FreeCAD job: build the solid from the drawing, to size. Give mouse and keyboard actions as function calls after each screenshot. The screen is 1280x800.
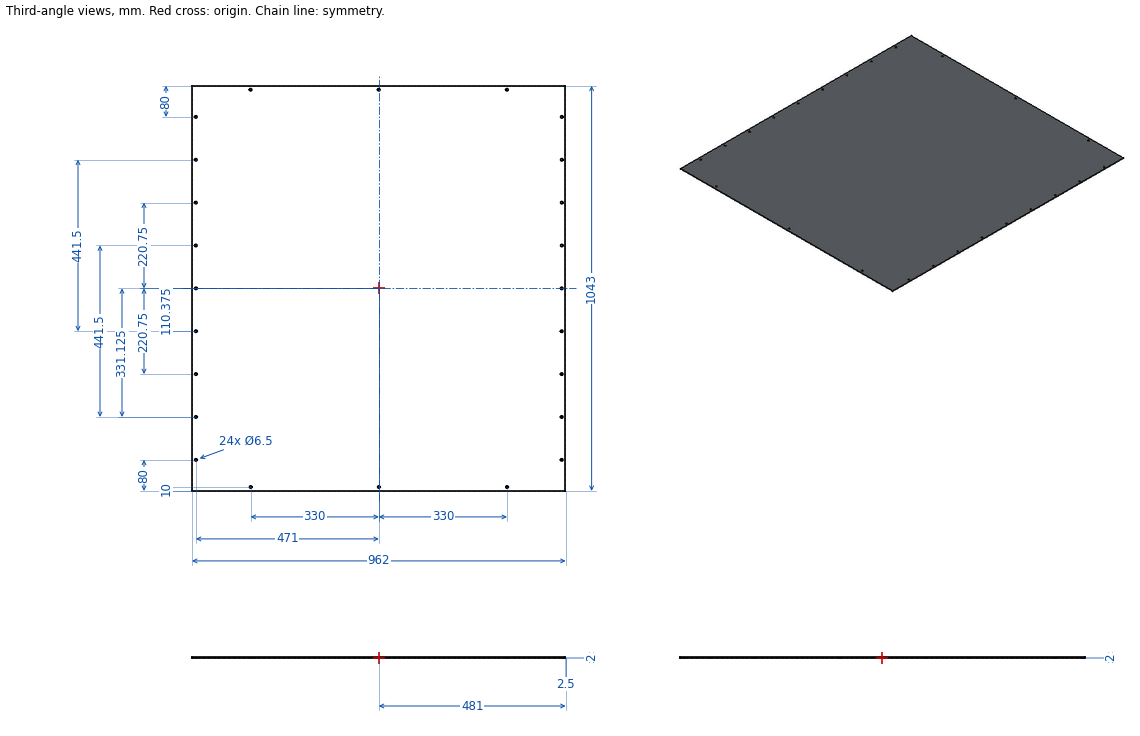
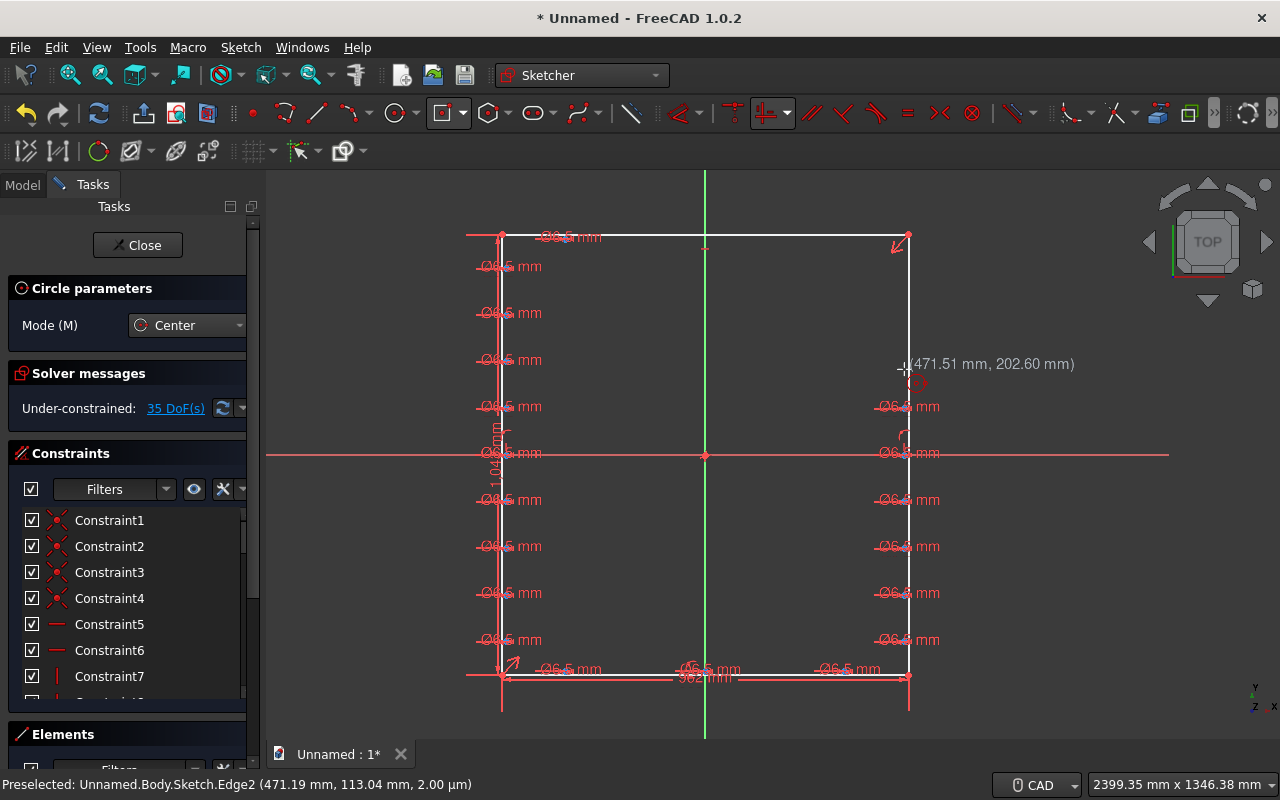
scroll(904, 362, up, 7)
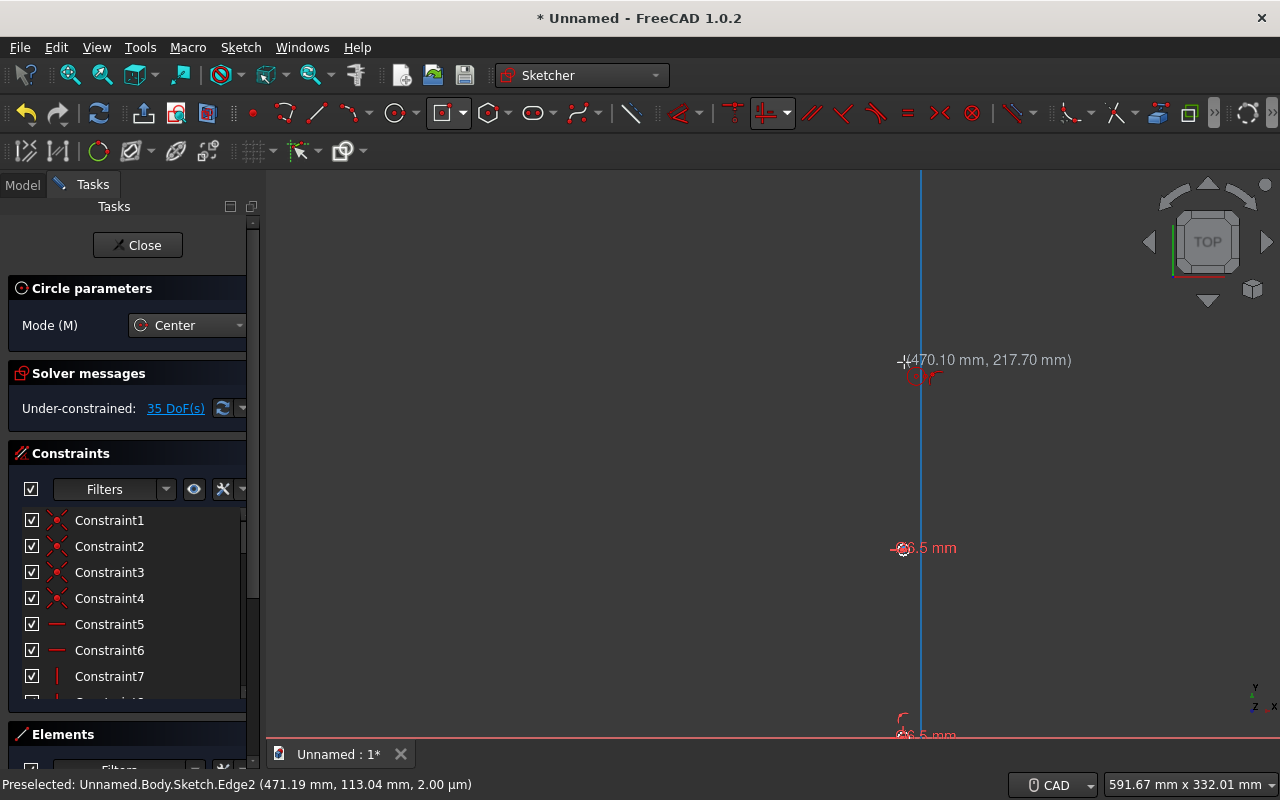
click(904, 360)
move(900, 356)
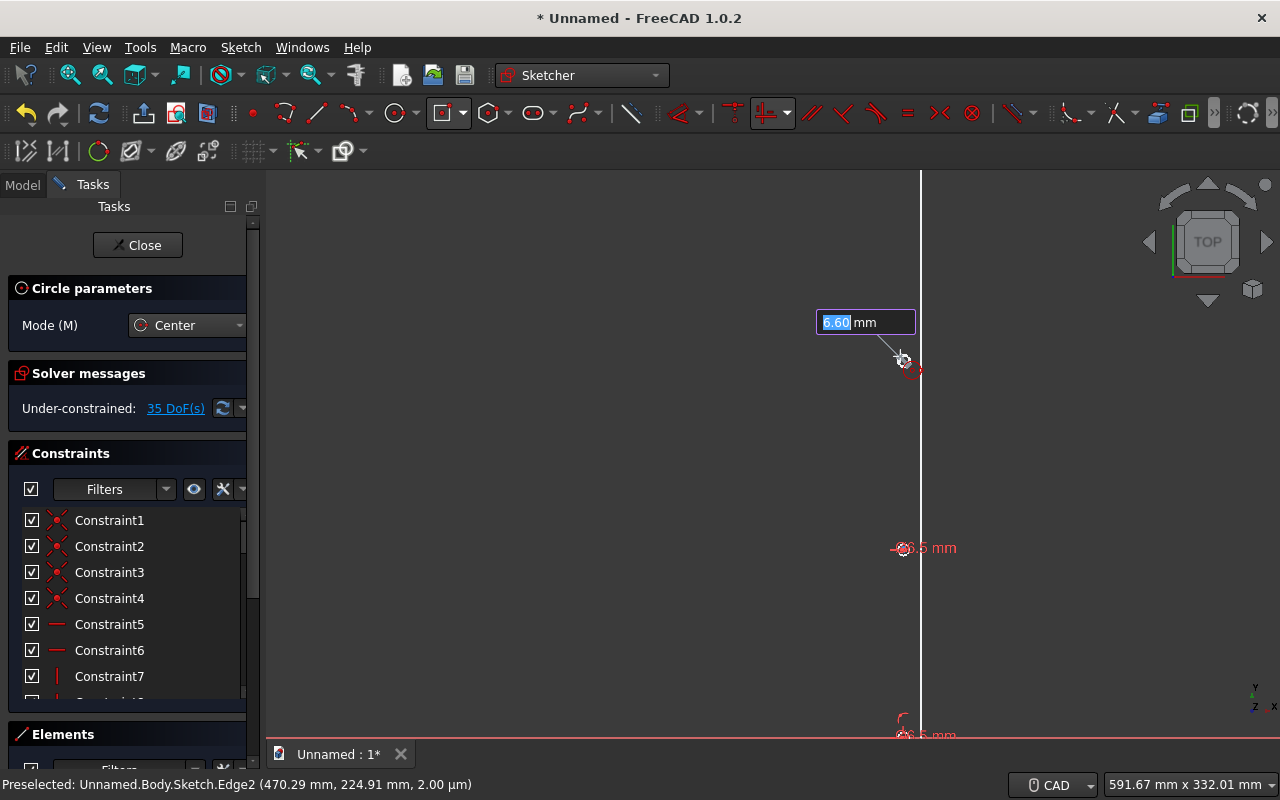
text(6.5)
key(Return)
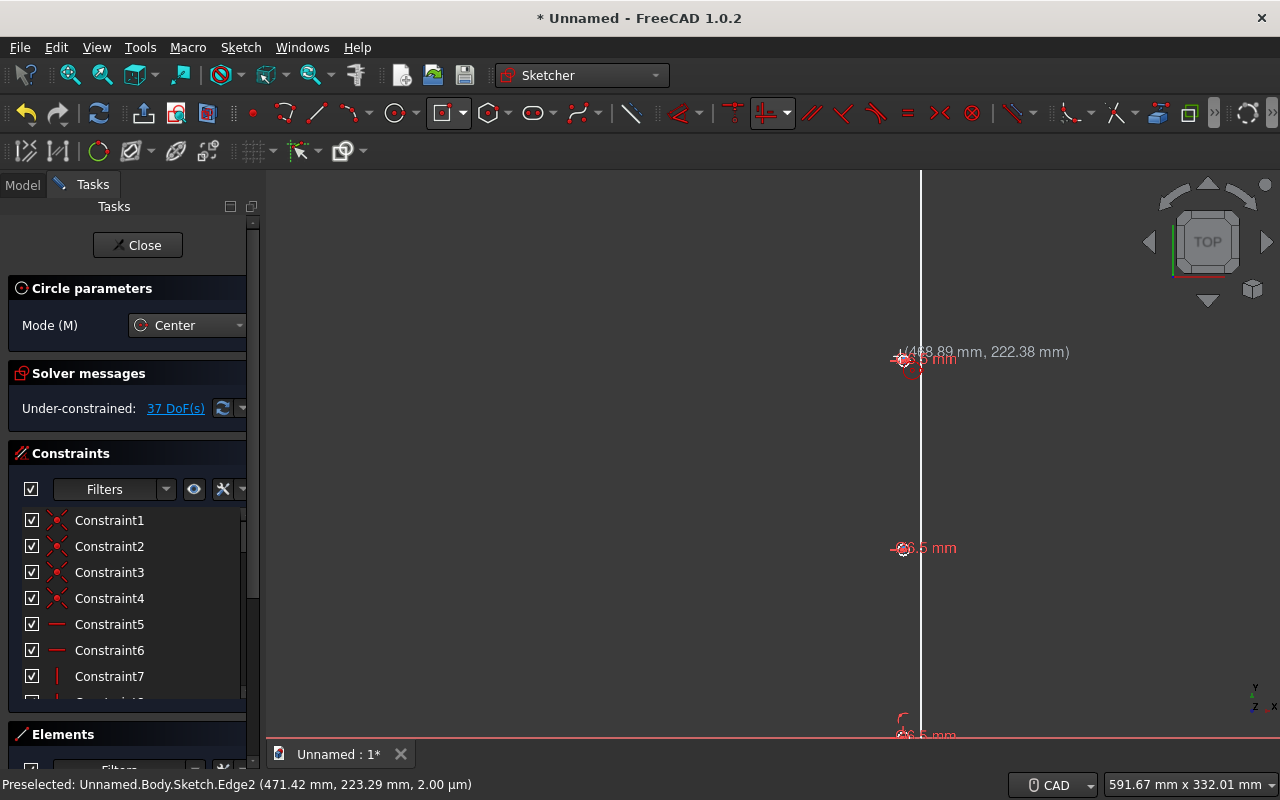
scroll(858, 383, down, 8)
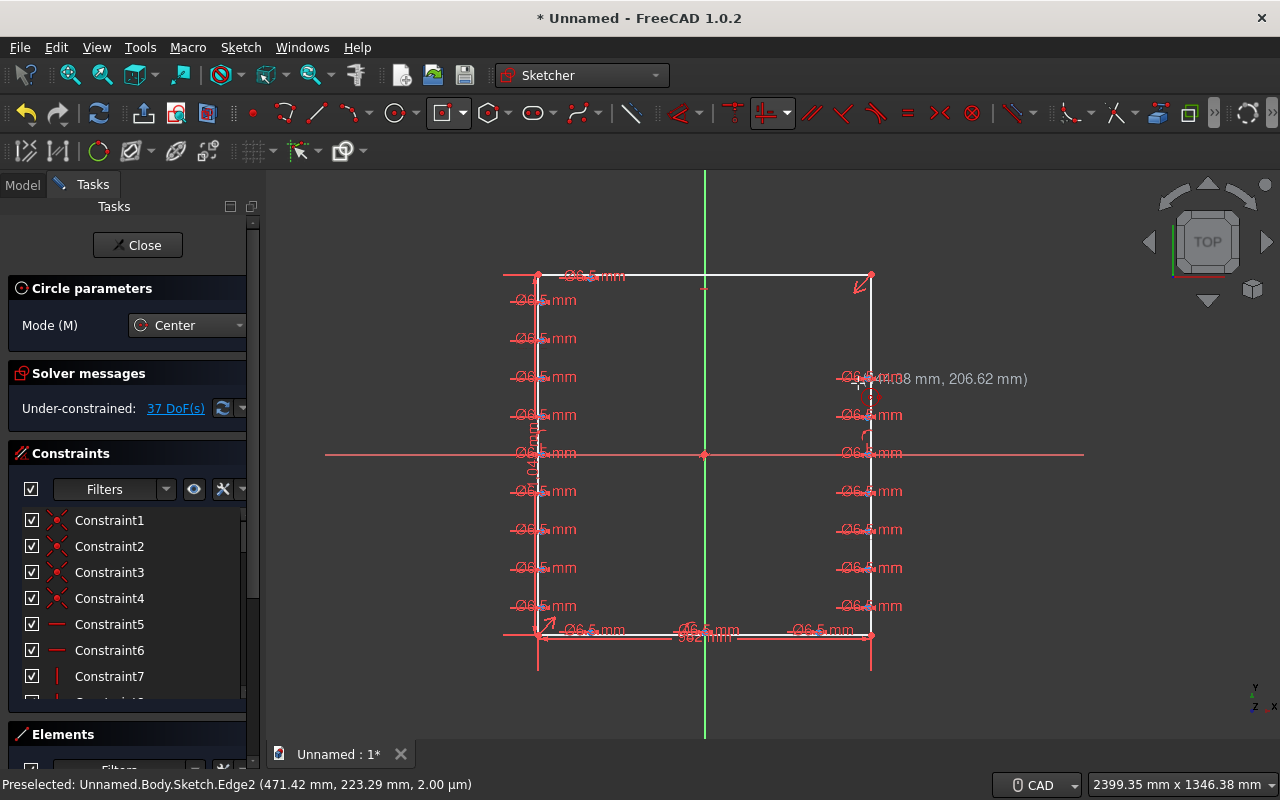
scroll(705, 278, up, 16)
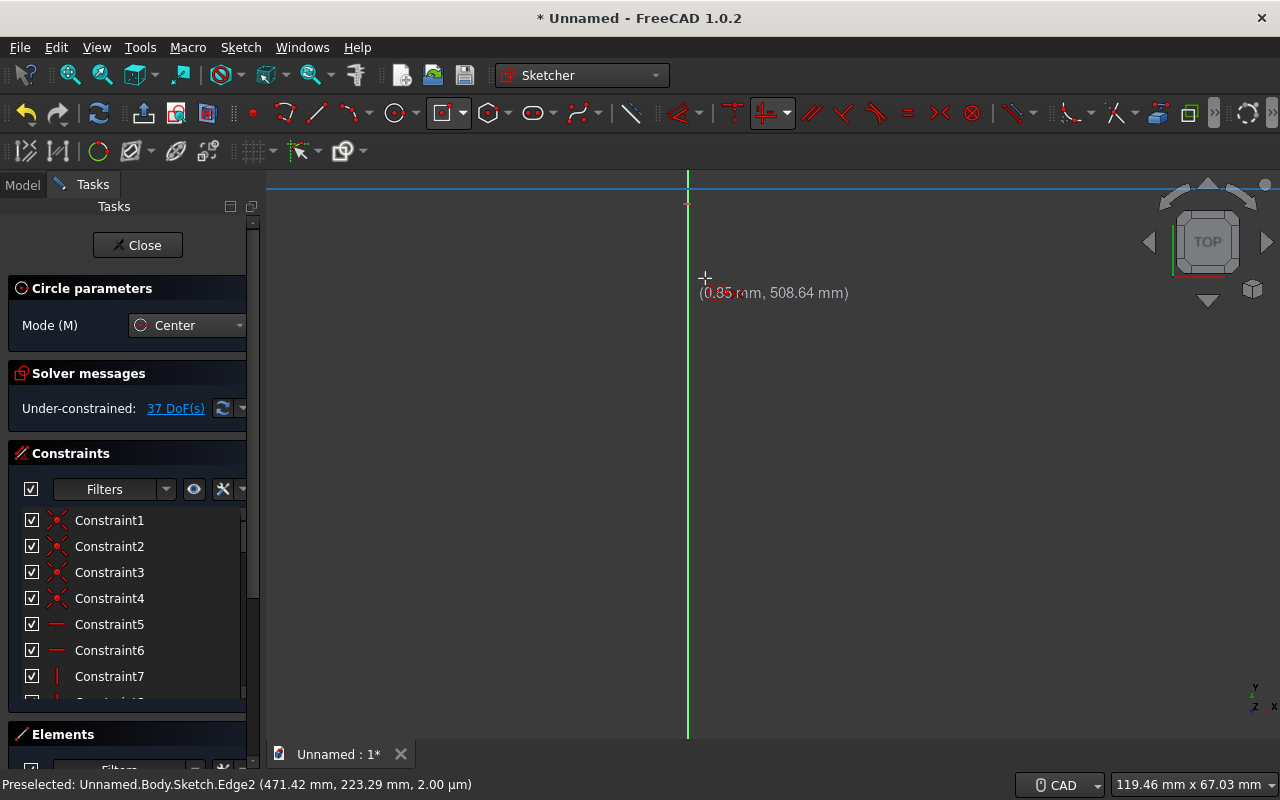
scroll(705, 236, down, 15)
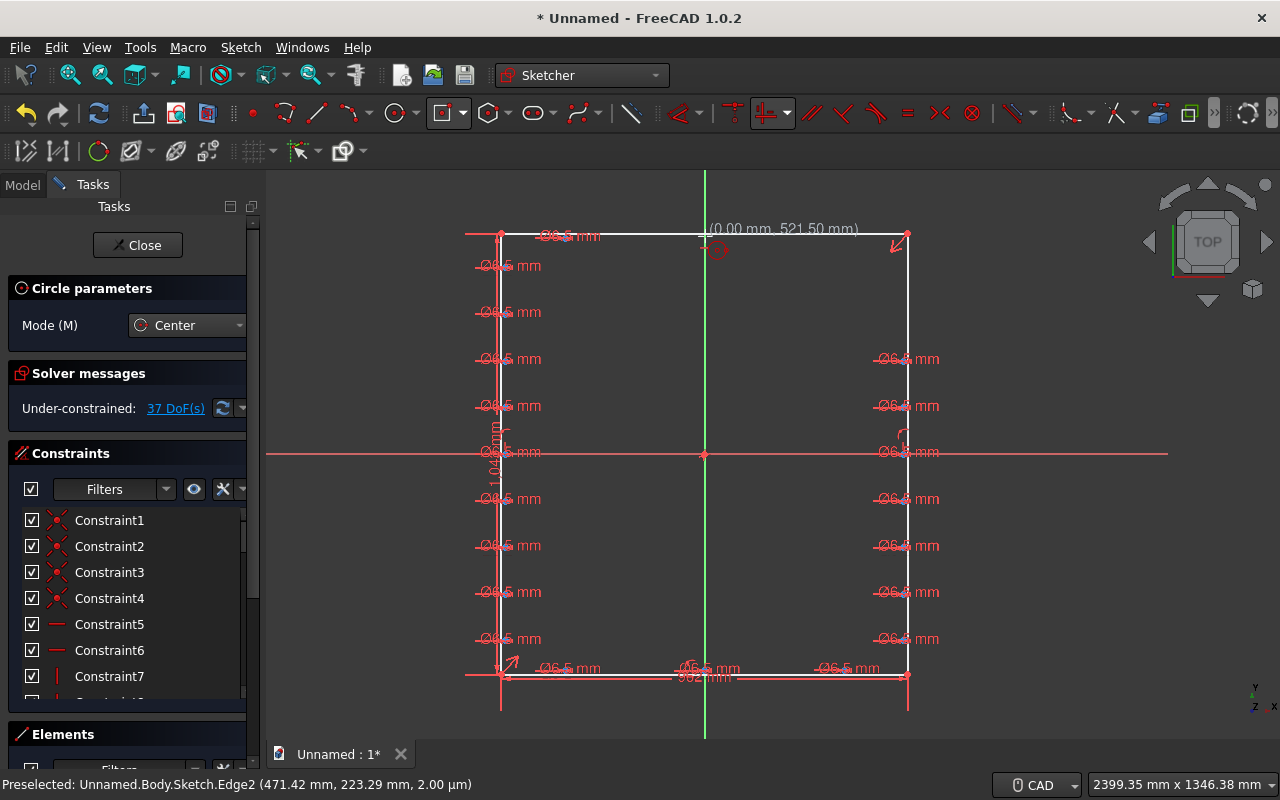
scroll(705, 238, up, 7)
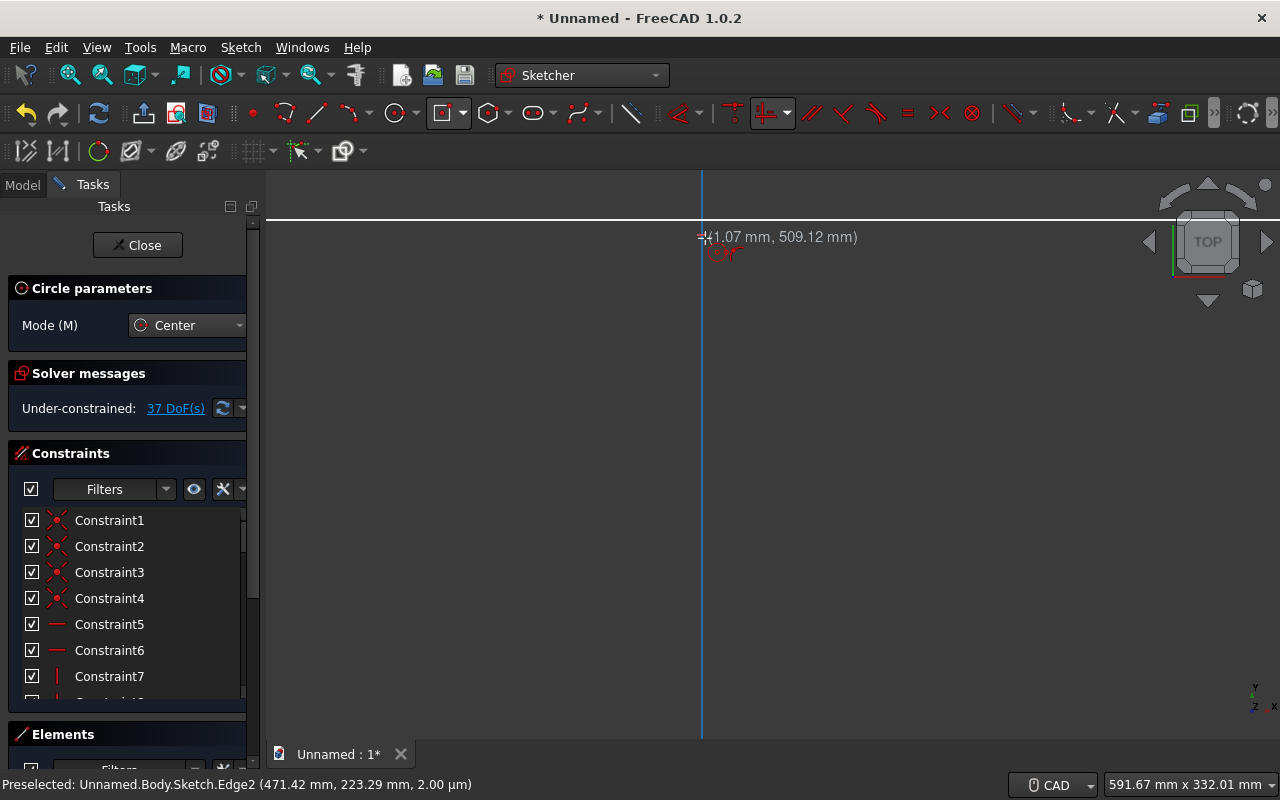
click(702, 238)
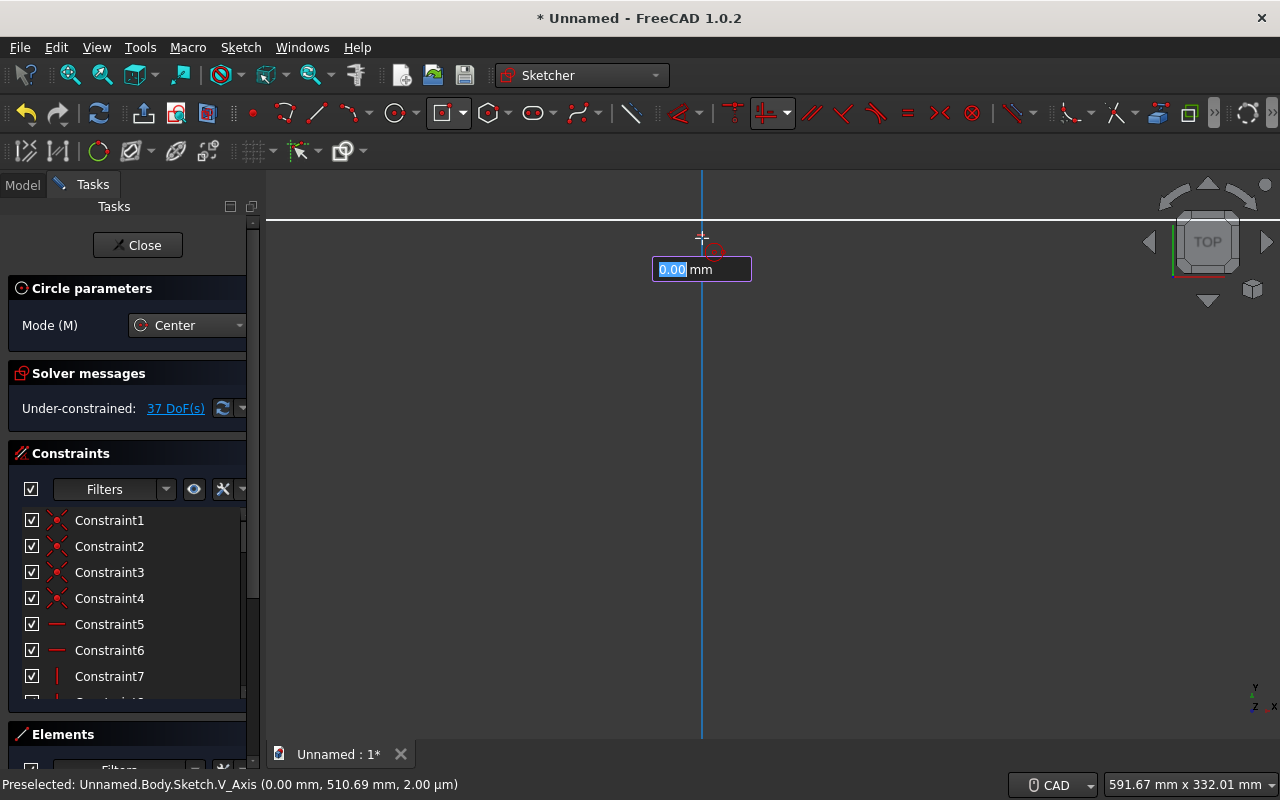
scroll(707, 236, up, 6)
move(706, 235)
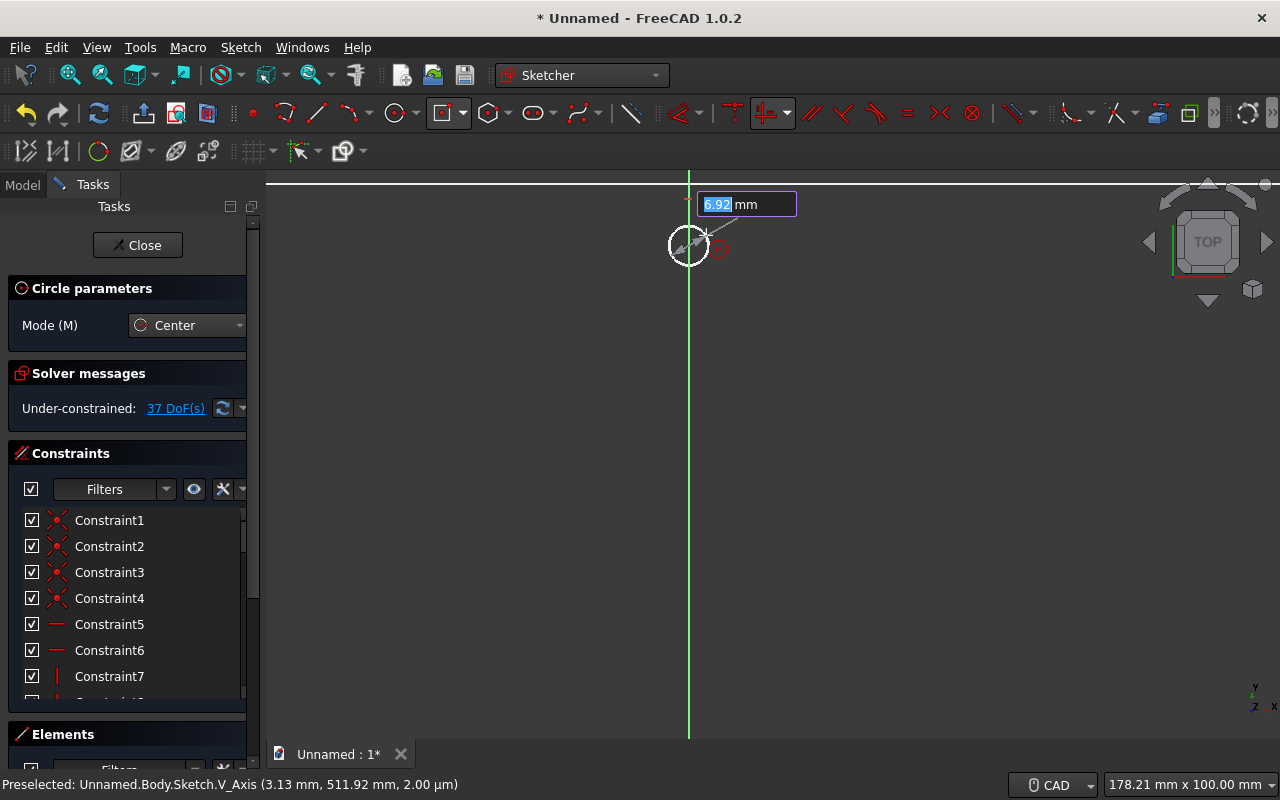
text(6.5)
key(Return)